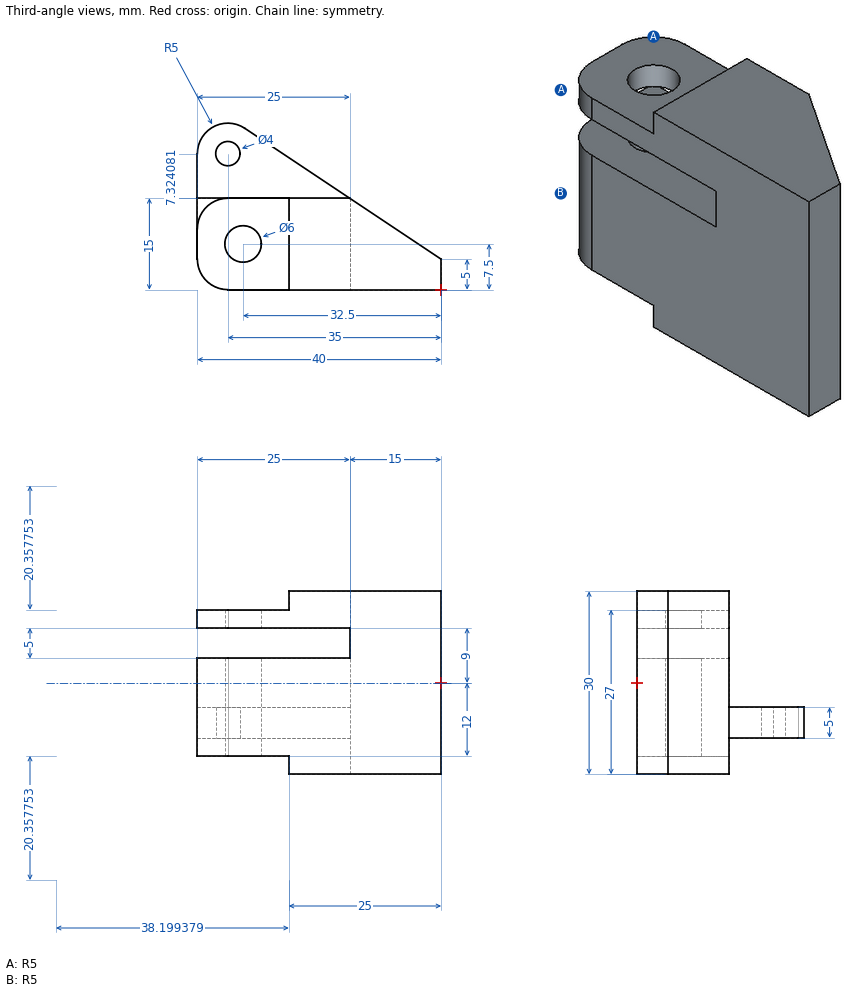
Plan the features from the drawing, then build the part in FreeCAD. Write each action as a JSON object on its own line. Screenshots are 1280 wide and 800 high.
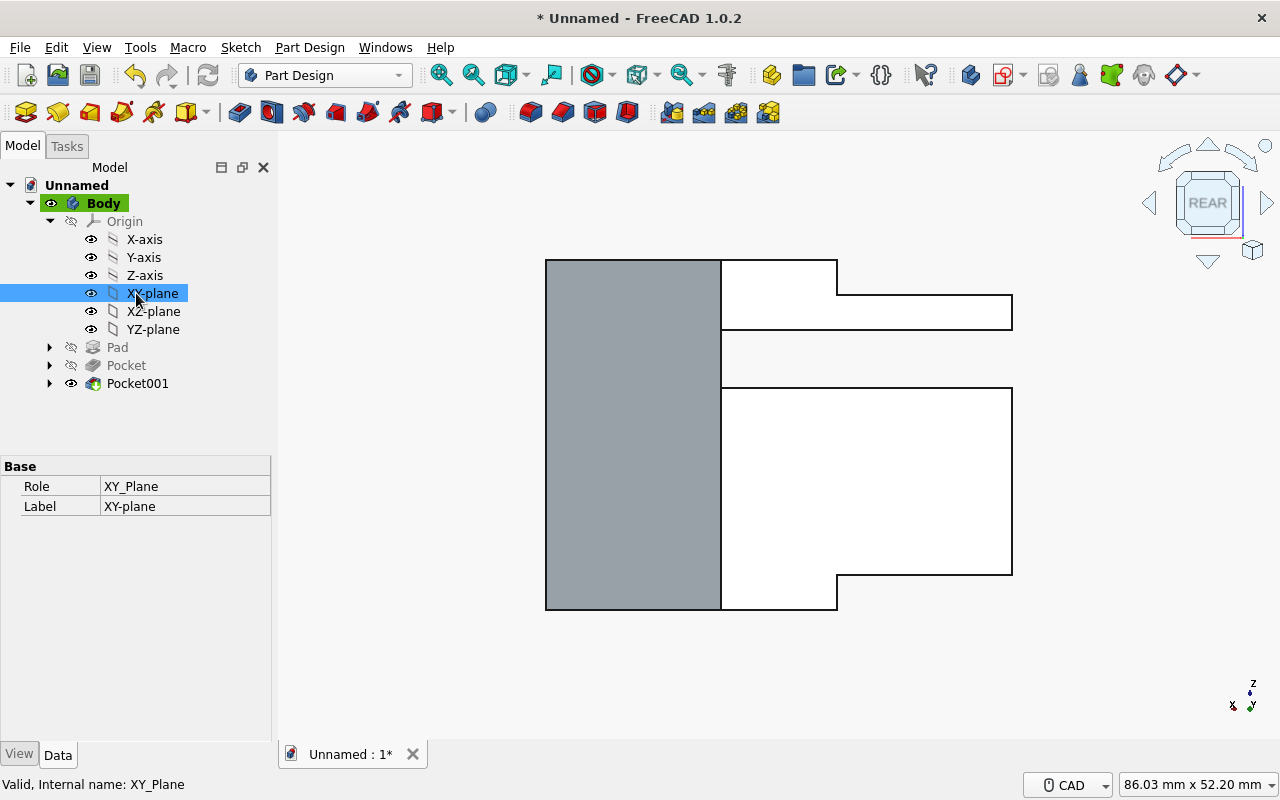
{"action": "left_click", "coordinate": [1176, 76]}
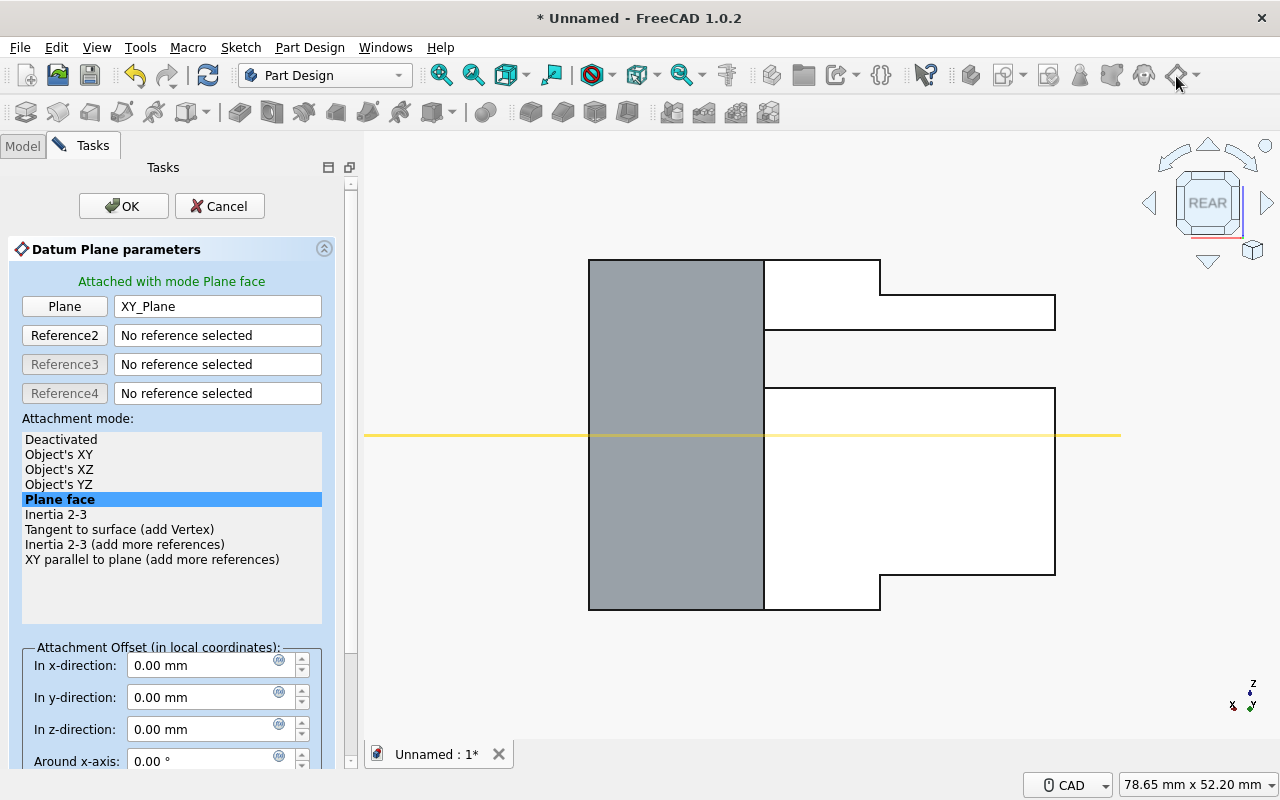
{"action": "triple_click", "coordinate": [210, 729]}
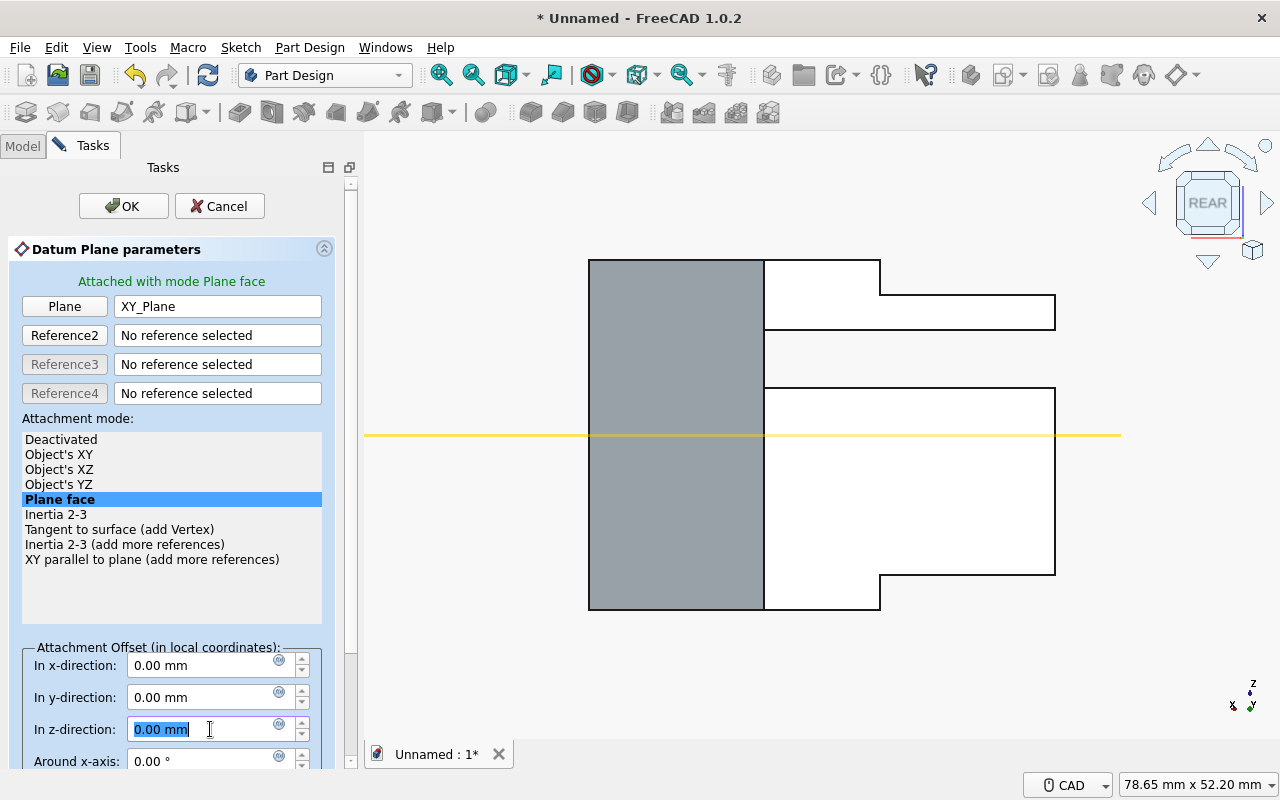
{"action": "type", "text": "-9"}
{"action": "key", "text": "Tab"}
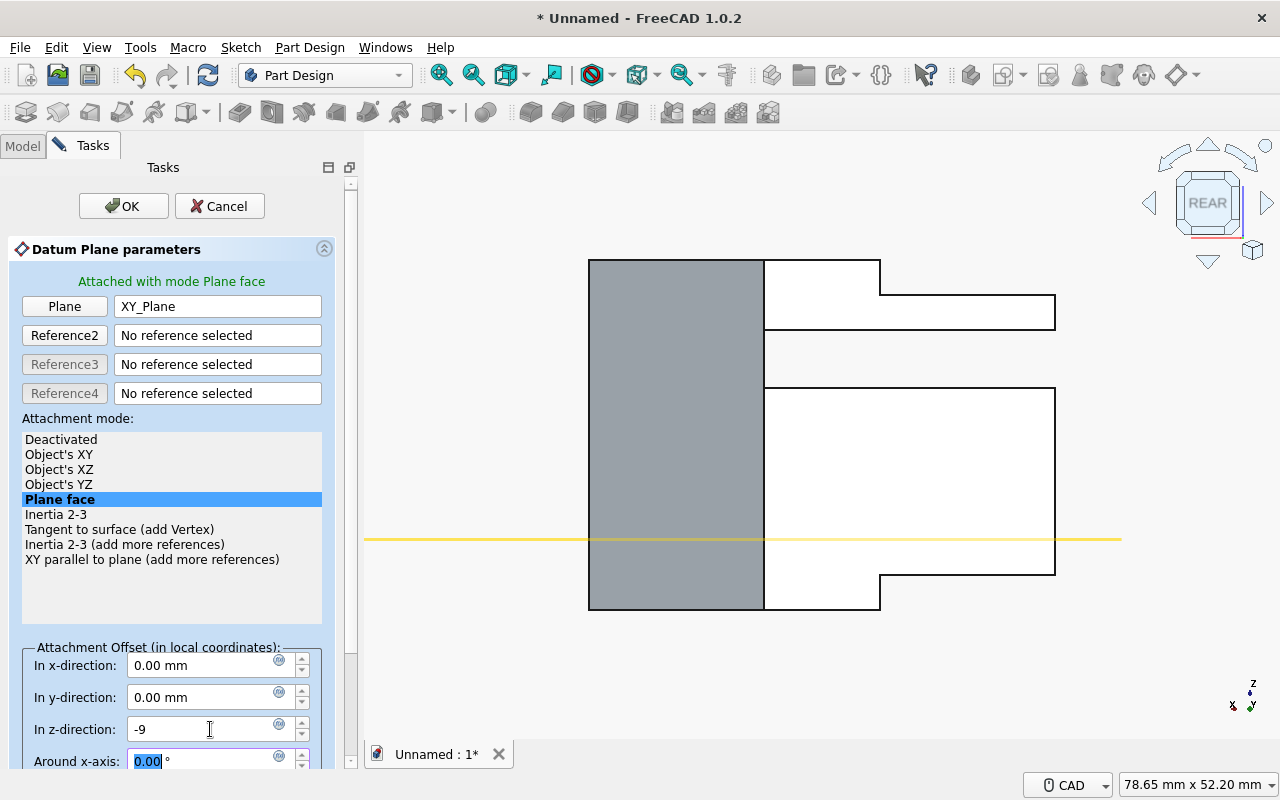
{"action": "left_click", "coordinate": [124, 206]}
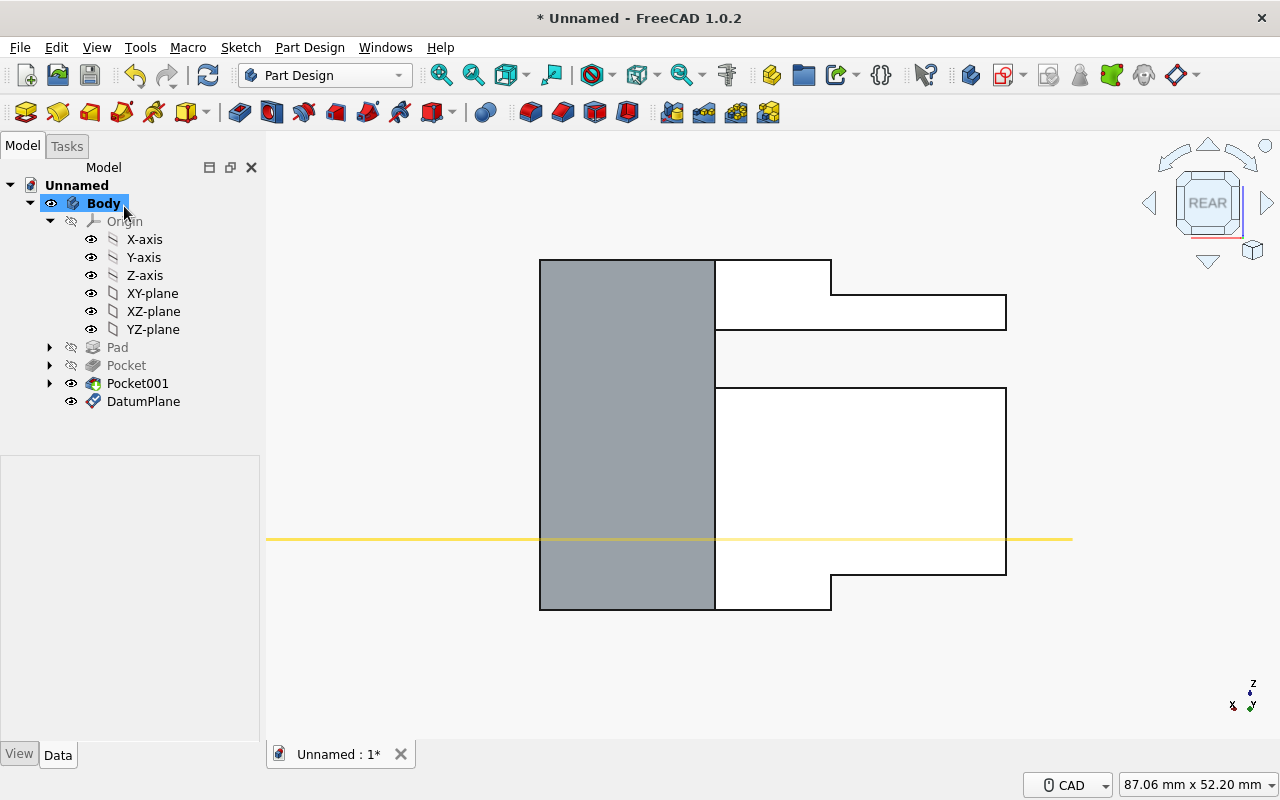
{"action": "left_click", "coordinate": [116, 401]}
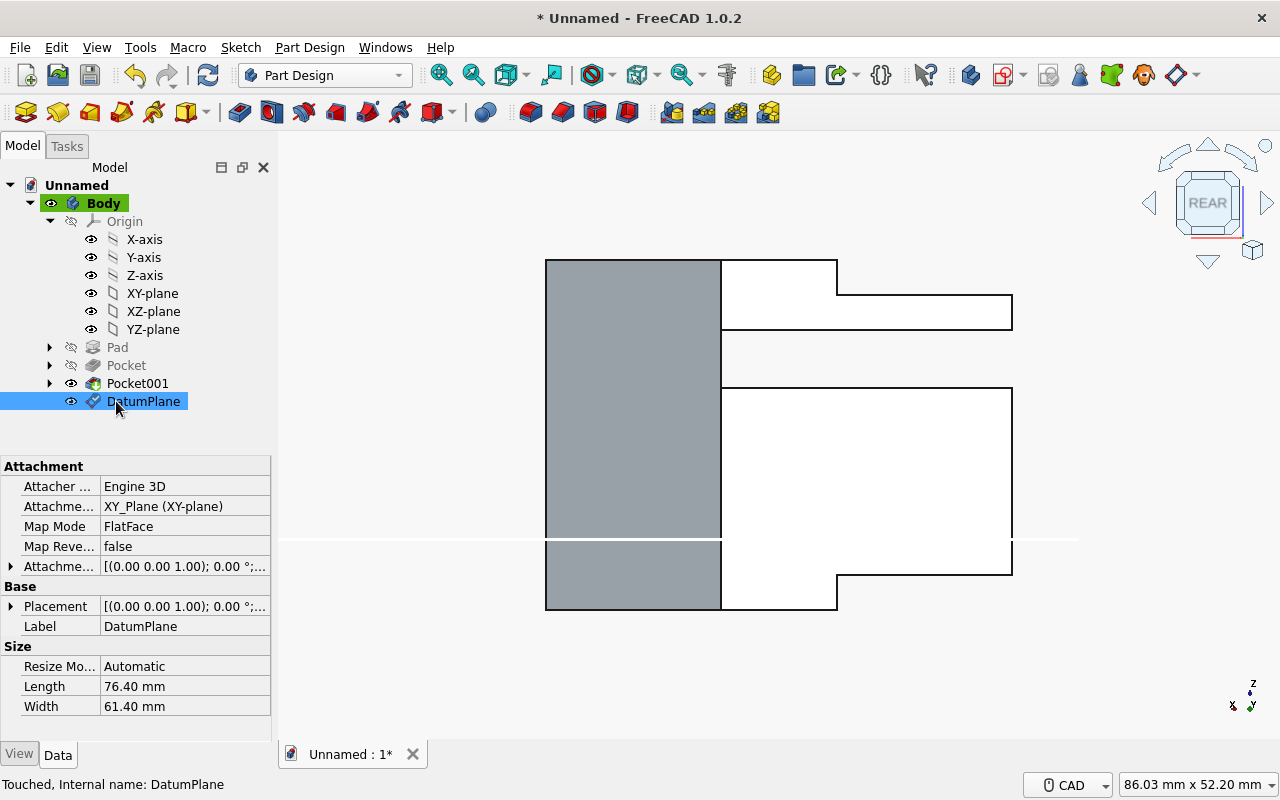
{"action": "left_click", "coordinate": [1004, 76]}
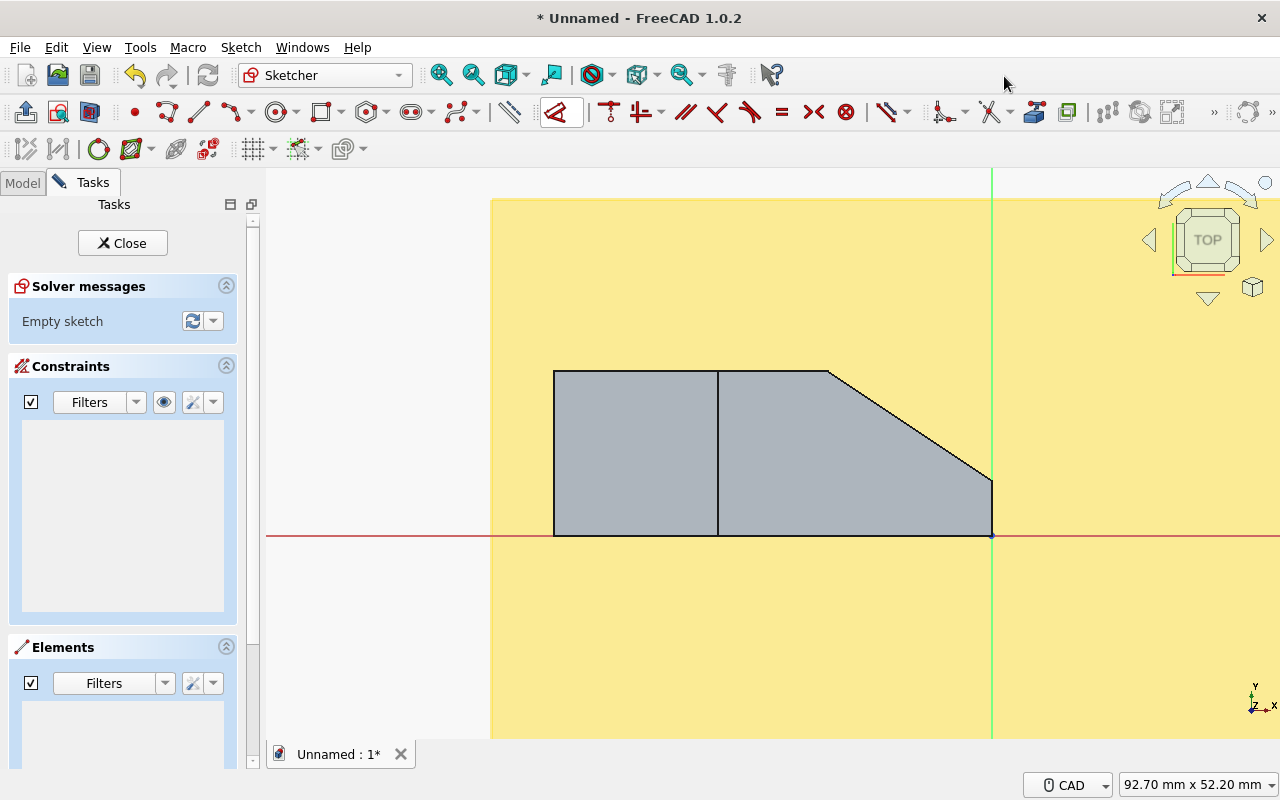
{"action": "key", "text": "q s"}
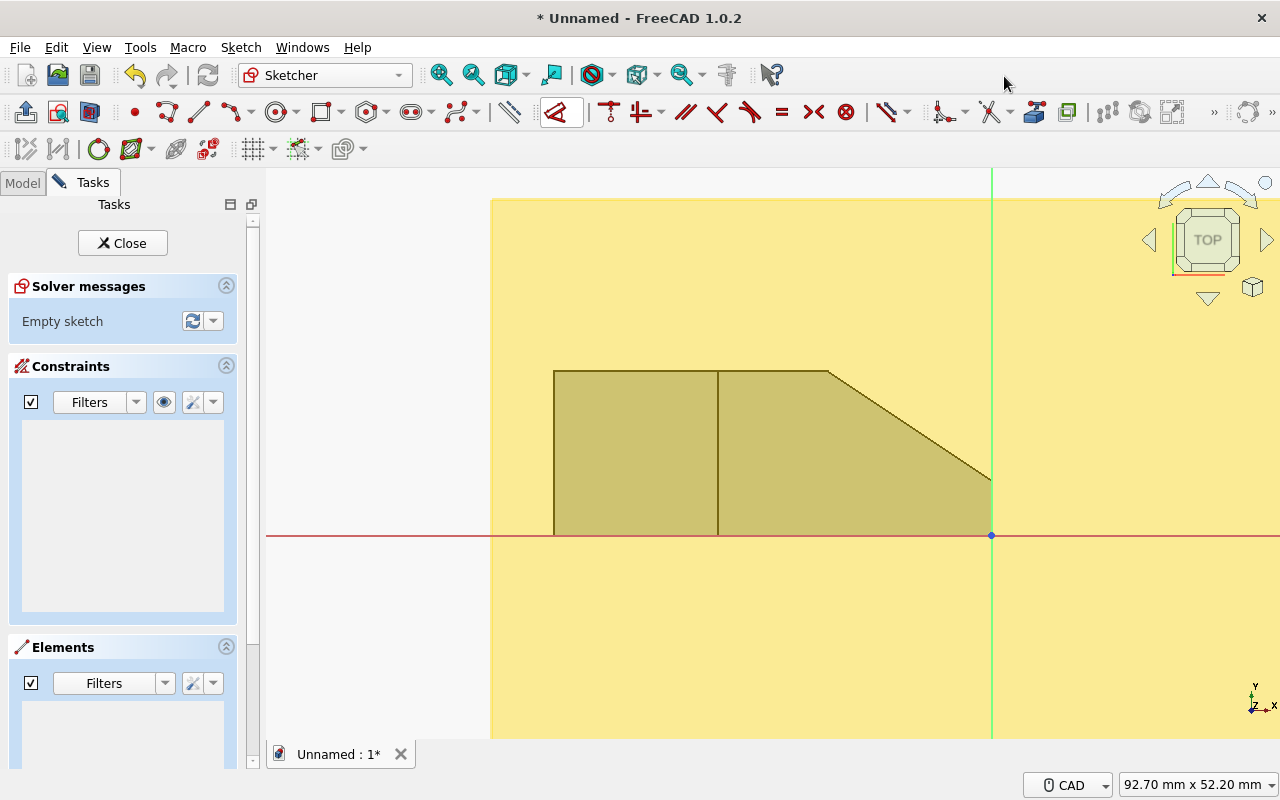
{"action": "key", "text": "g m"}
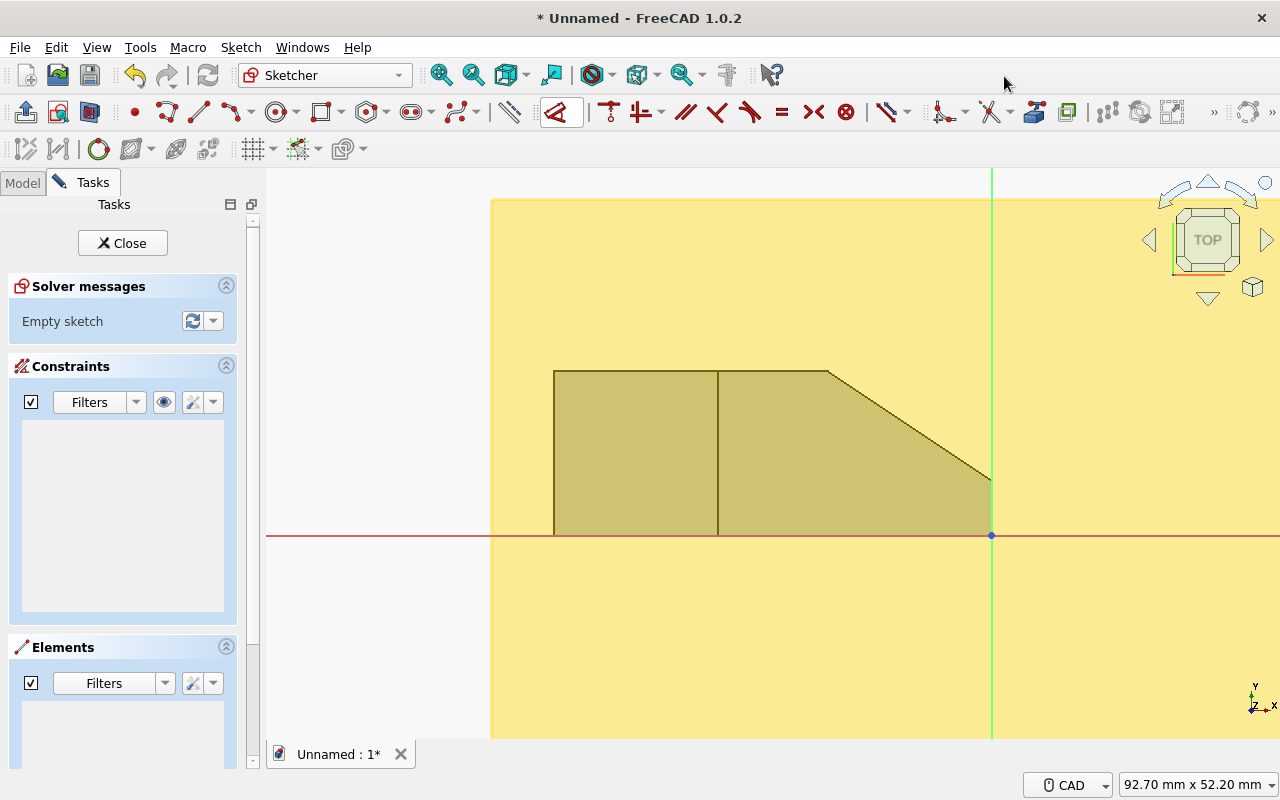
{"action": "left_click", "coordinate": [554, 291]}
{"action": "left_click", "coordinate": [554, 371]}
{"action": "left_click", "coordinate": [828, 371]}
{"action": "left_click", "coordinate": [639, 246]}
{"action": "right_click", "coordinate": [639, 246]}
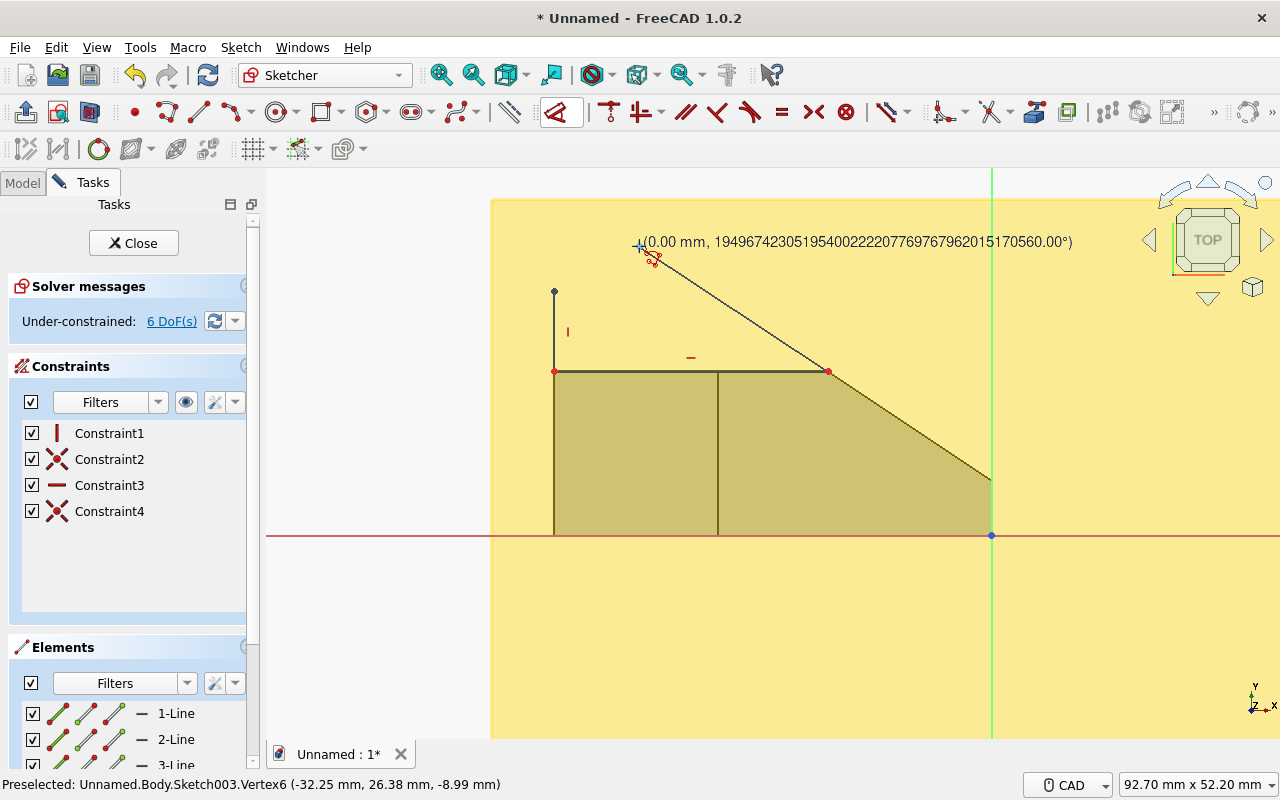
{"action": "left_click", "coordinate": [232, 112]}